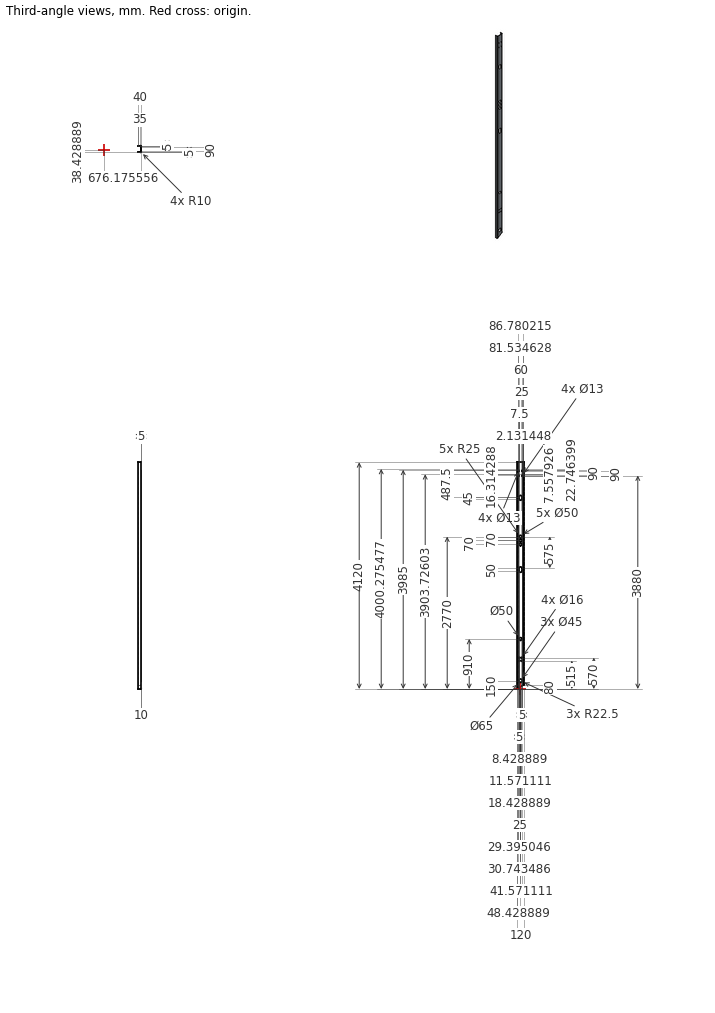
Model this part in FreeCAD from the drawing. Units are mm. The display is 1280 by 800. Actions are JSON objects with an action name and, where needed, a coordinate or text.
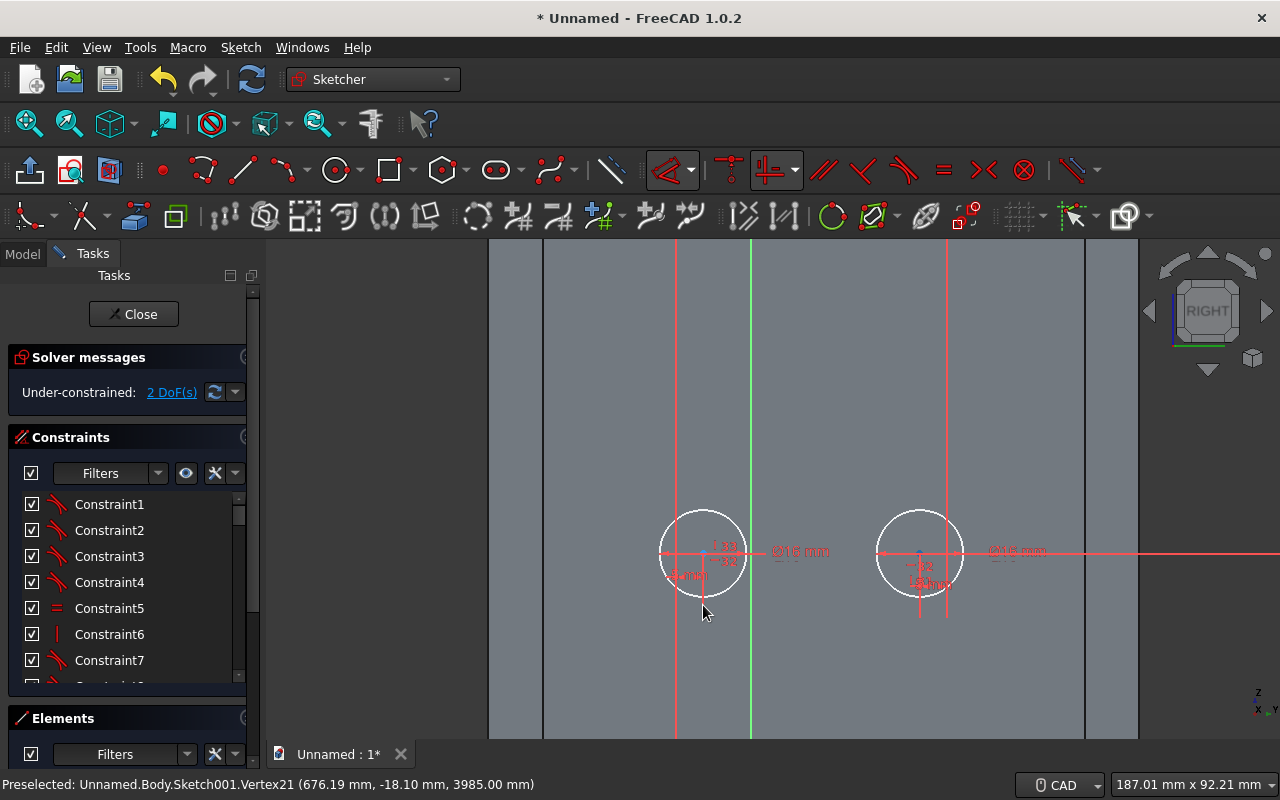
{"action": "left_click", "coordinate": [703, 554]}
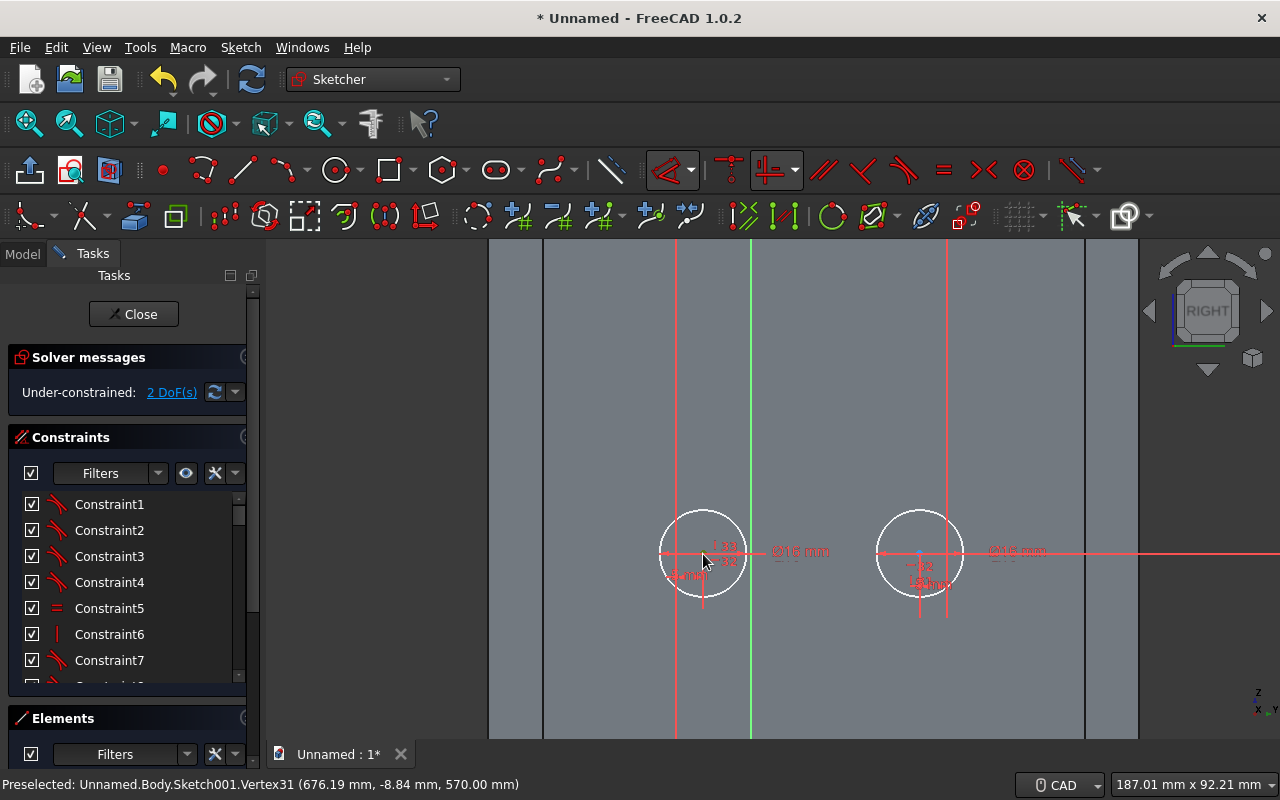
{"action": "key", "text": "l"}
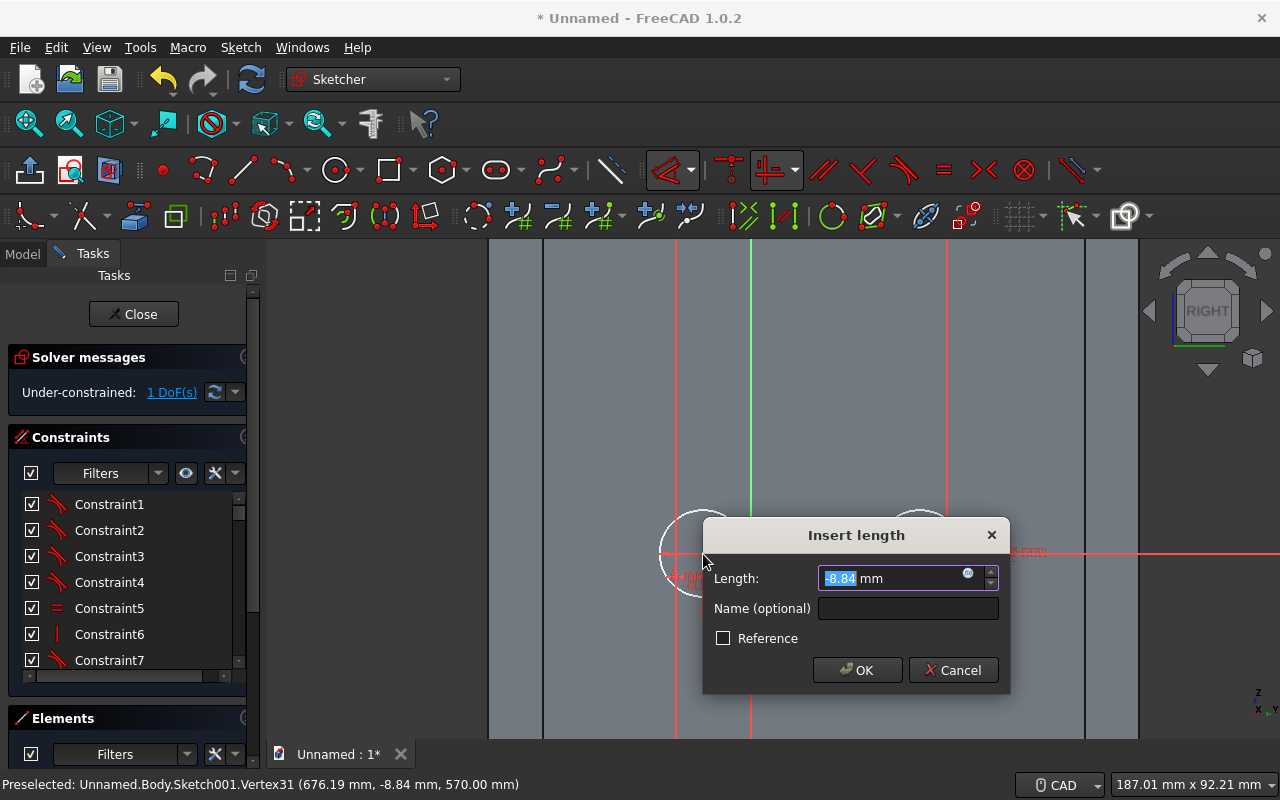
{"action": "type", "text": "-8.428889"}
{"action": "key", "text": "Return"}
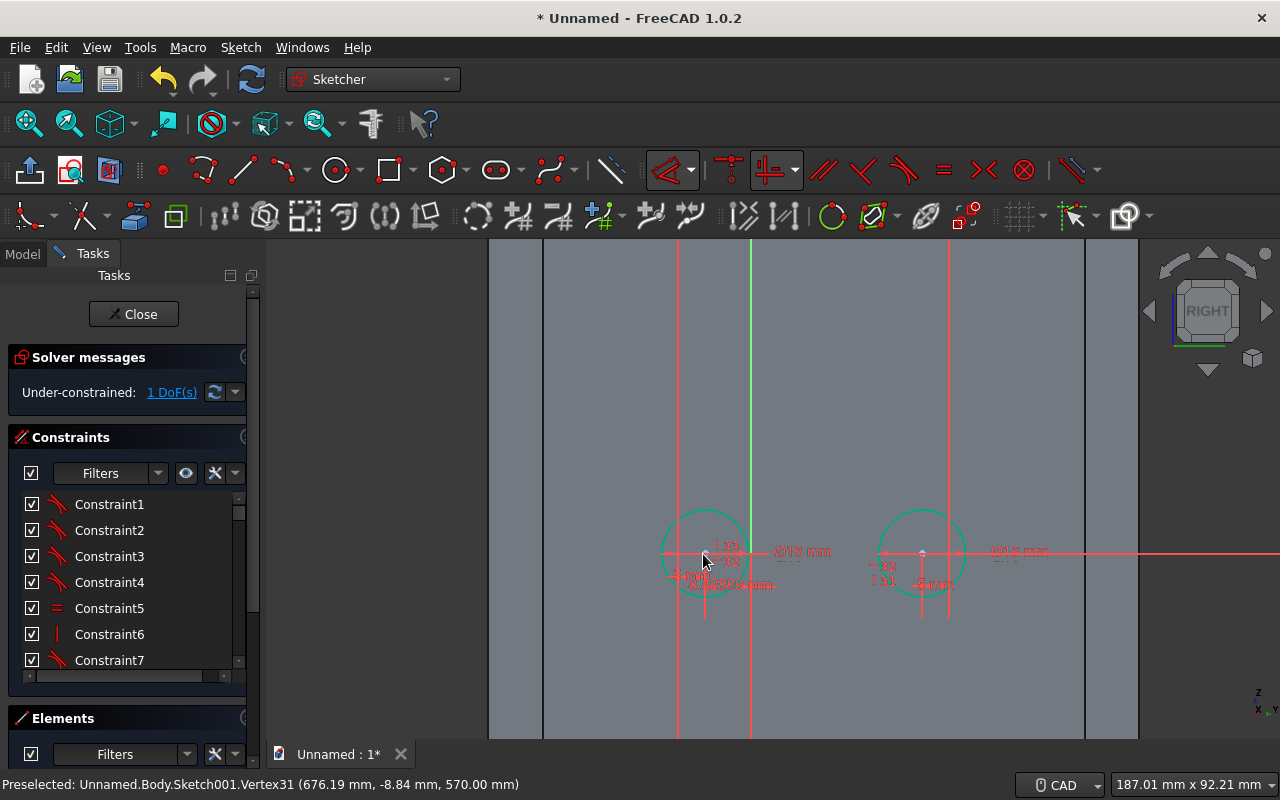
{"action": "scroll", "coordinate": [704, 489], "scroll_direction": "down", "scroll_amount": 15}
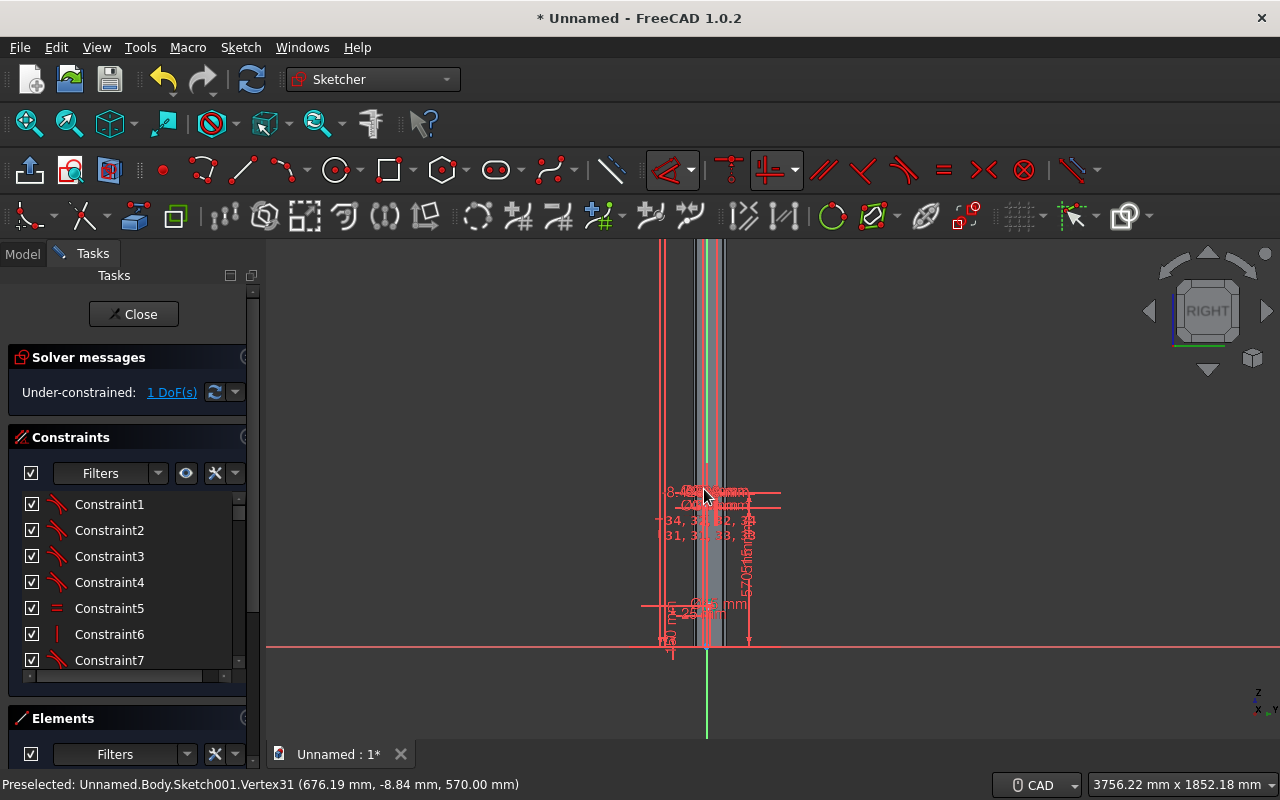
{"action": "scroll", "coordinate": [702, 653], "scroll_direction": "down", "scroll_amount": 6}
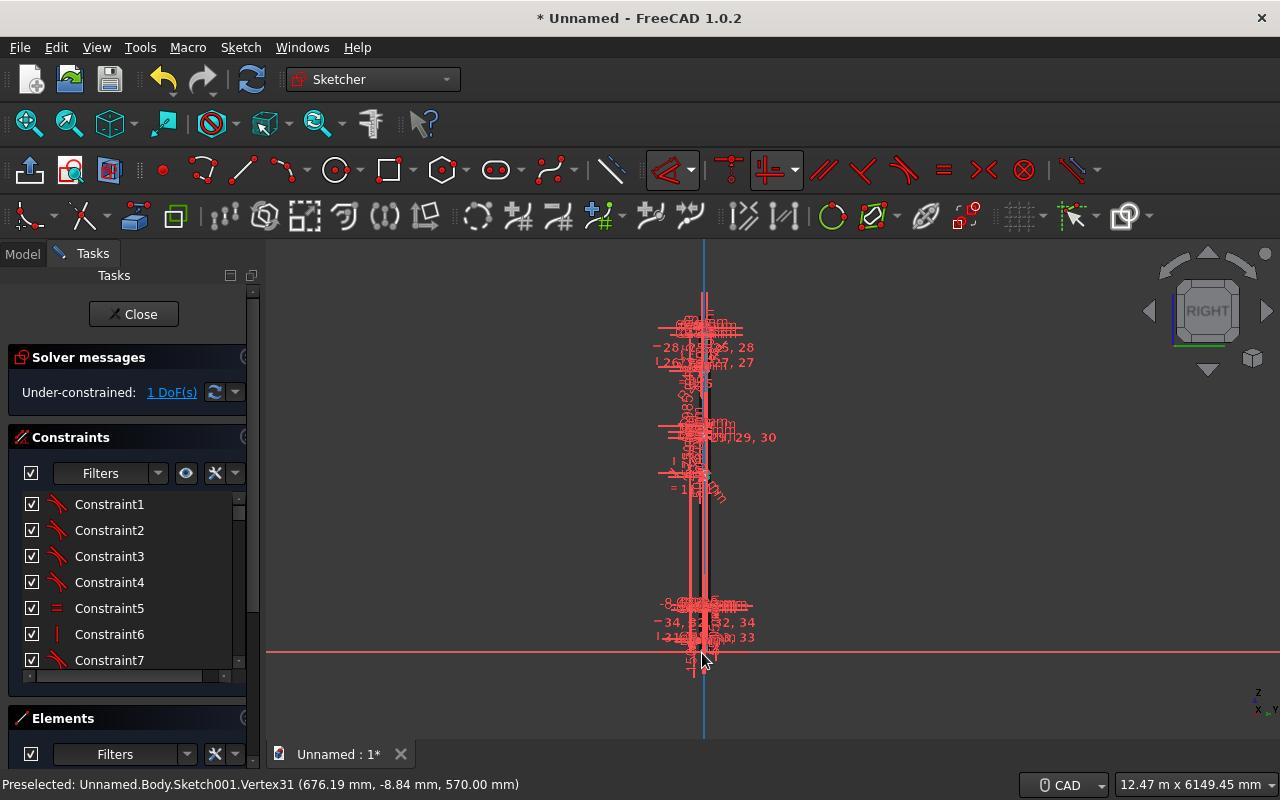
{"action": "scroll", "coordinate": [702, 328], "scroll_direction": "up", "scroll_amount": 17}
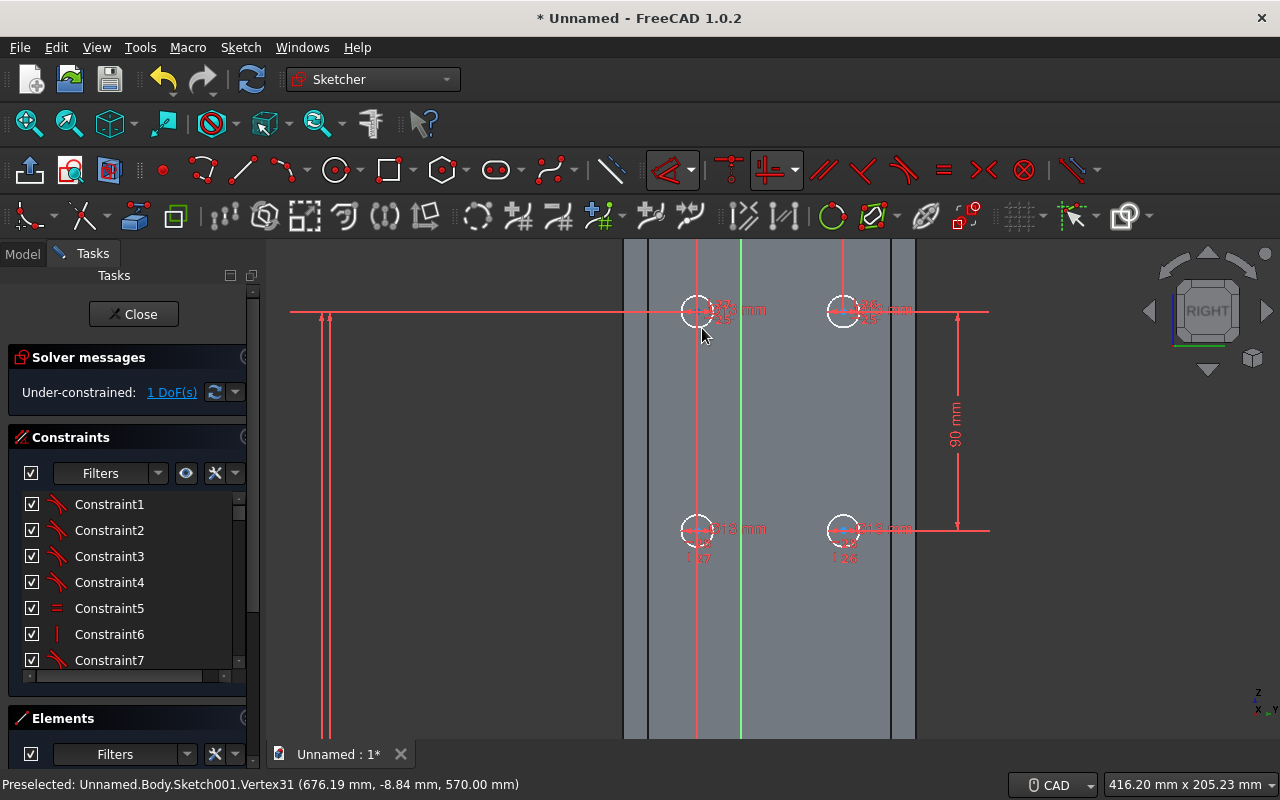
{"action": "left_click", "coordinate": [697, 312]}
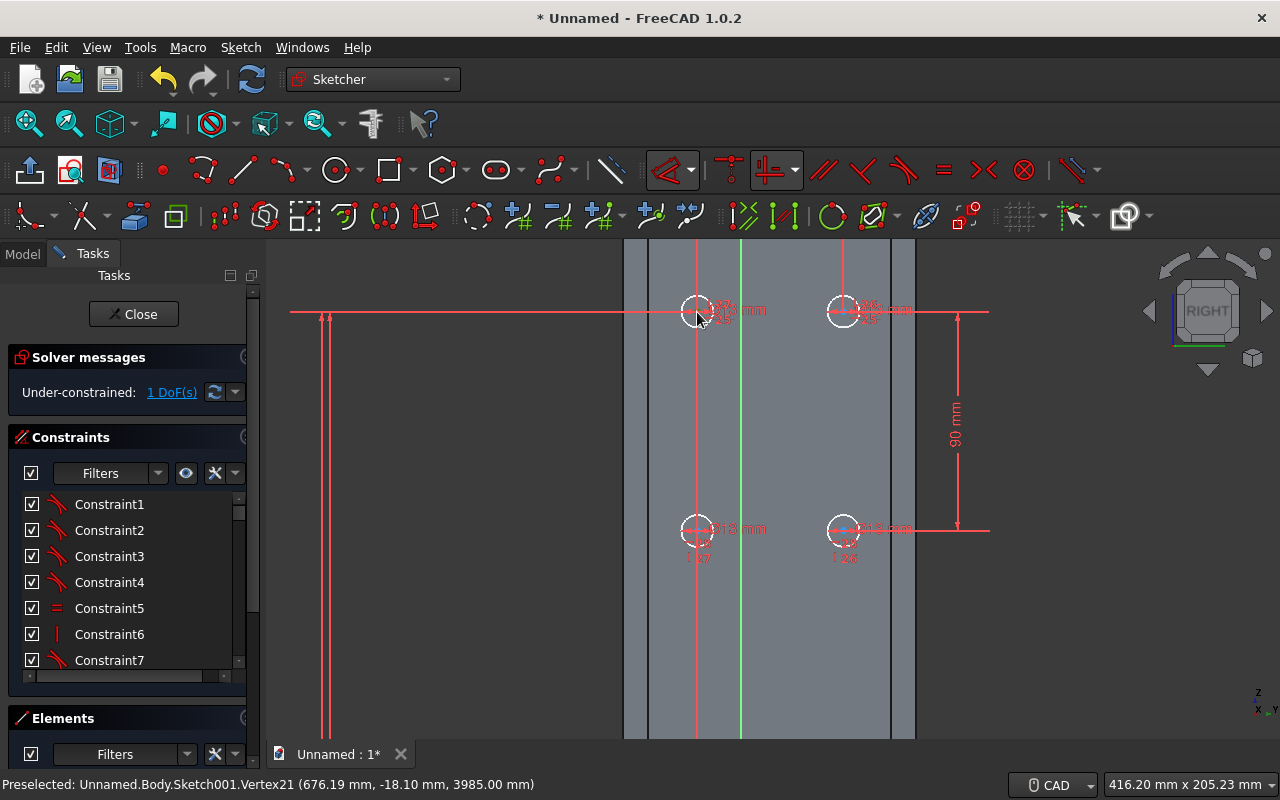
{"action": "key", "text": "l"}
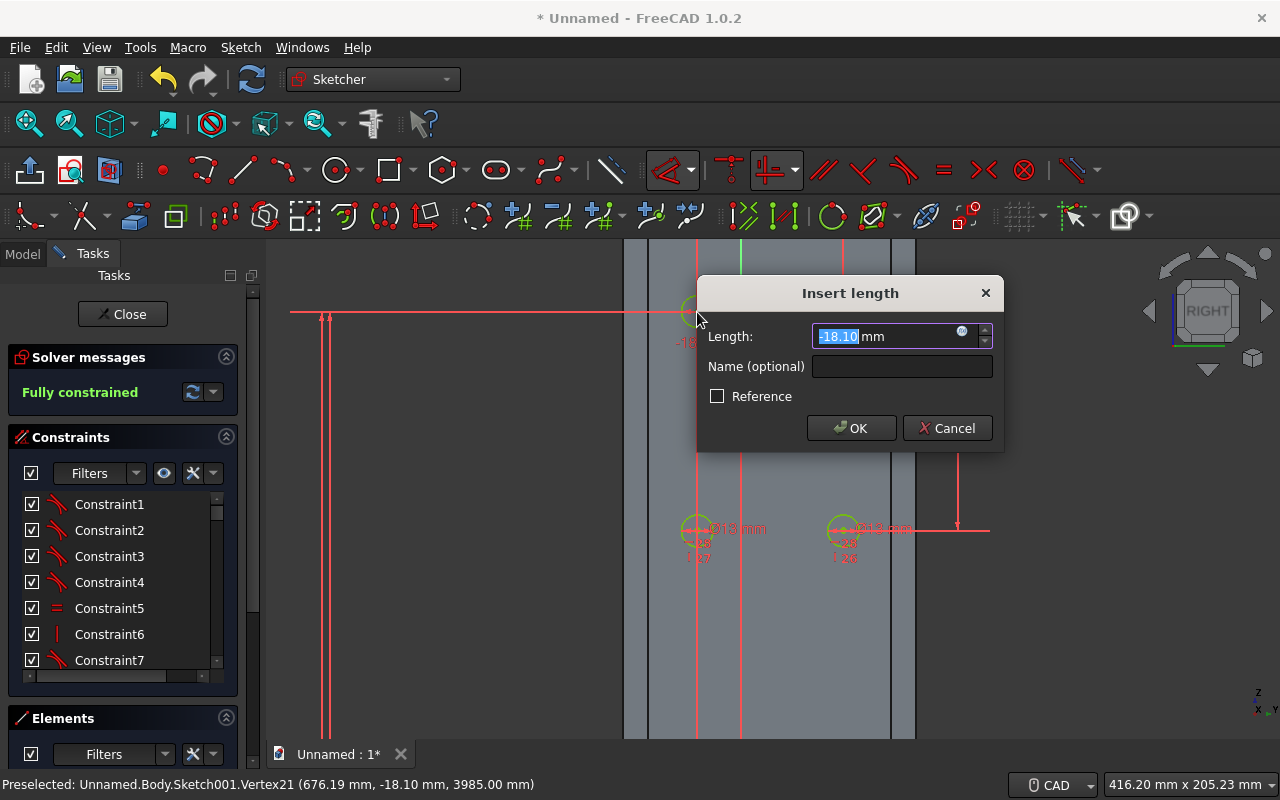
{"action": "type", "text": "-18.428889"}
{"action": "key", "text": "Return"}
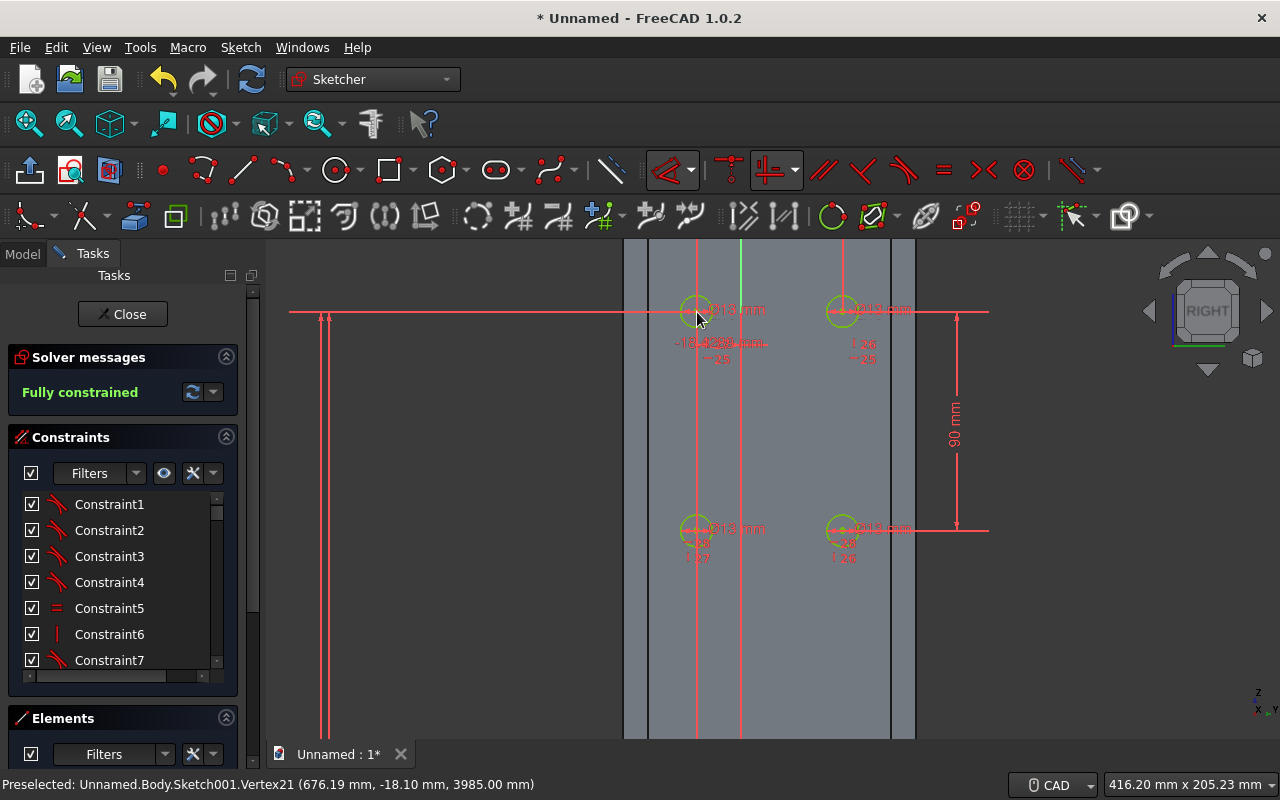
{"action": "left_click", "coordinate": [123, 314]}